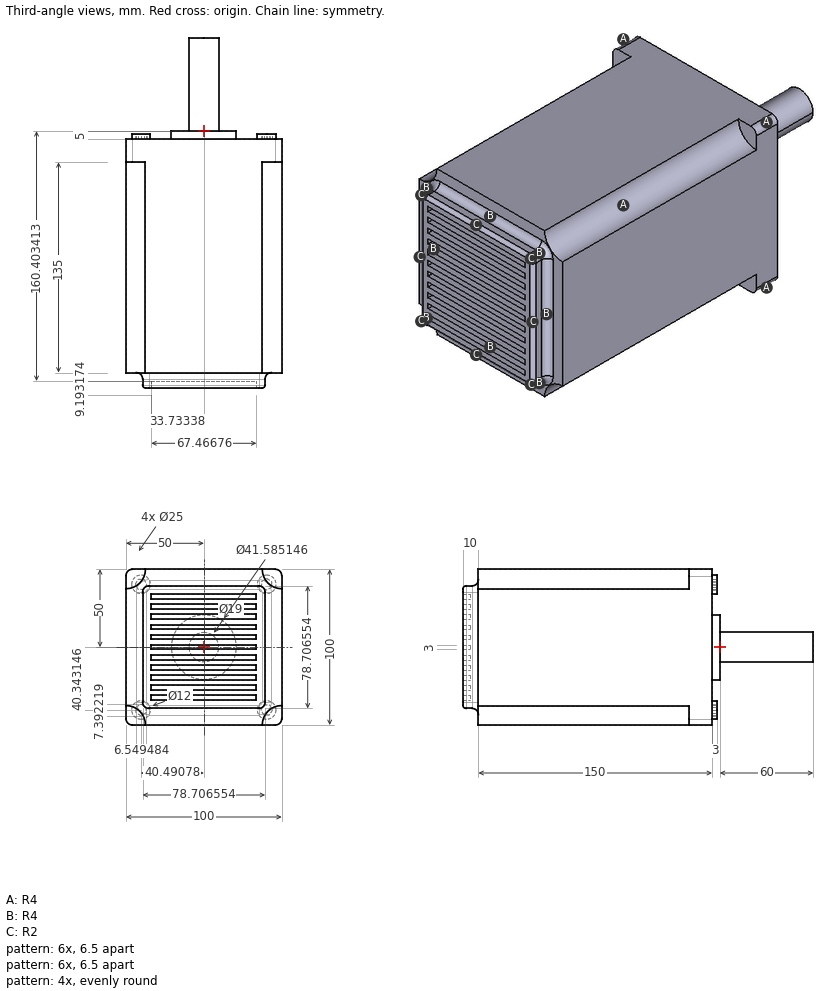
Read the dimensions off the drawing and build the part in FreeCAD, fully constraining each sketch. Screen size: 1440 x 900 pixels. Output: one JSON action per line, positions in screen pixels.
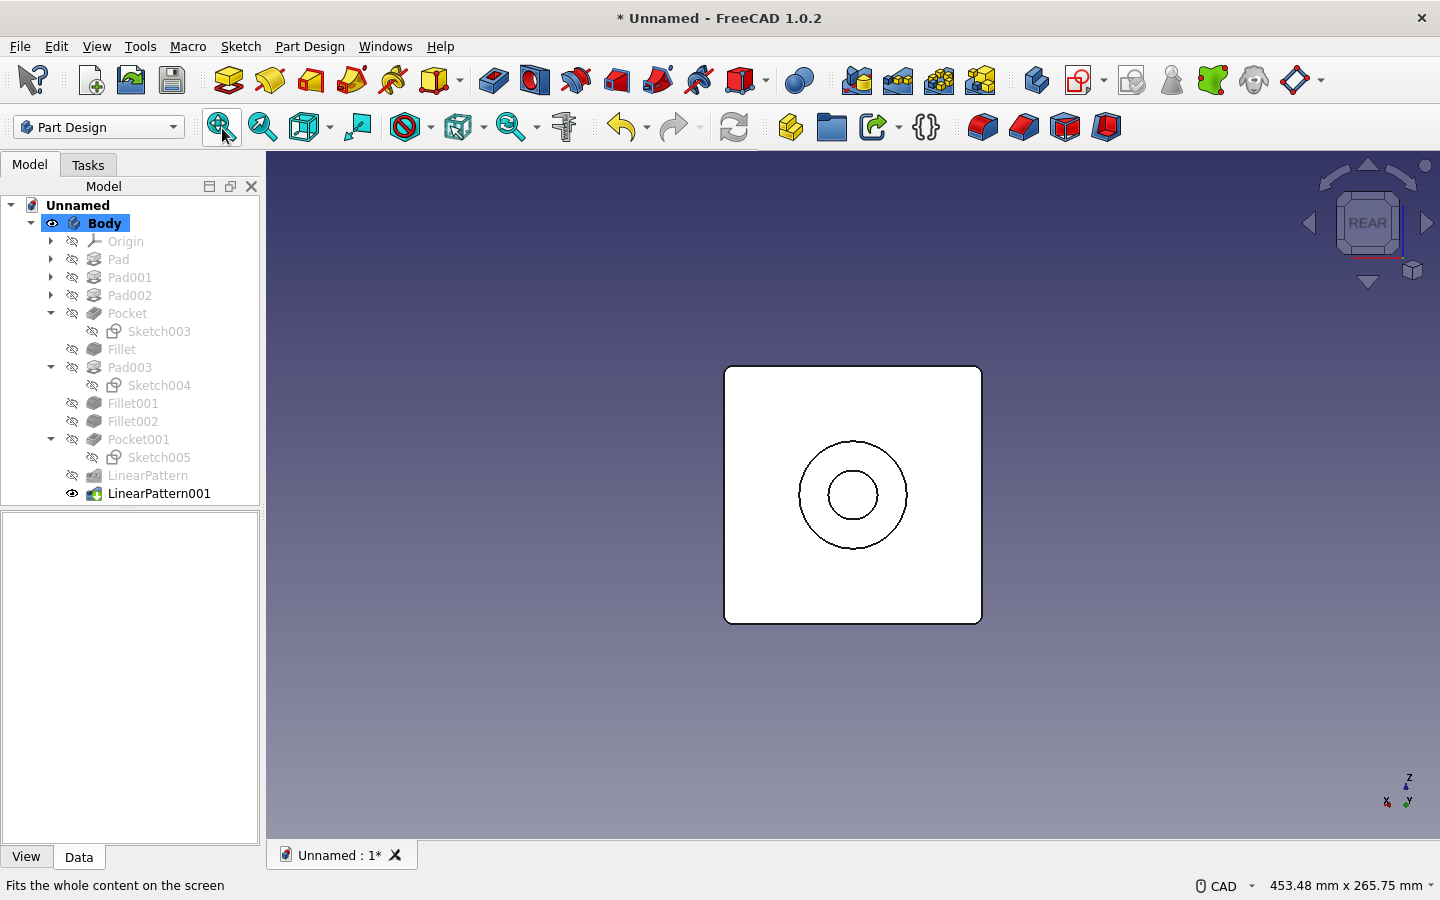
{"action": "left_click", "coordinate": [779, 568]}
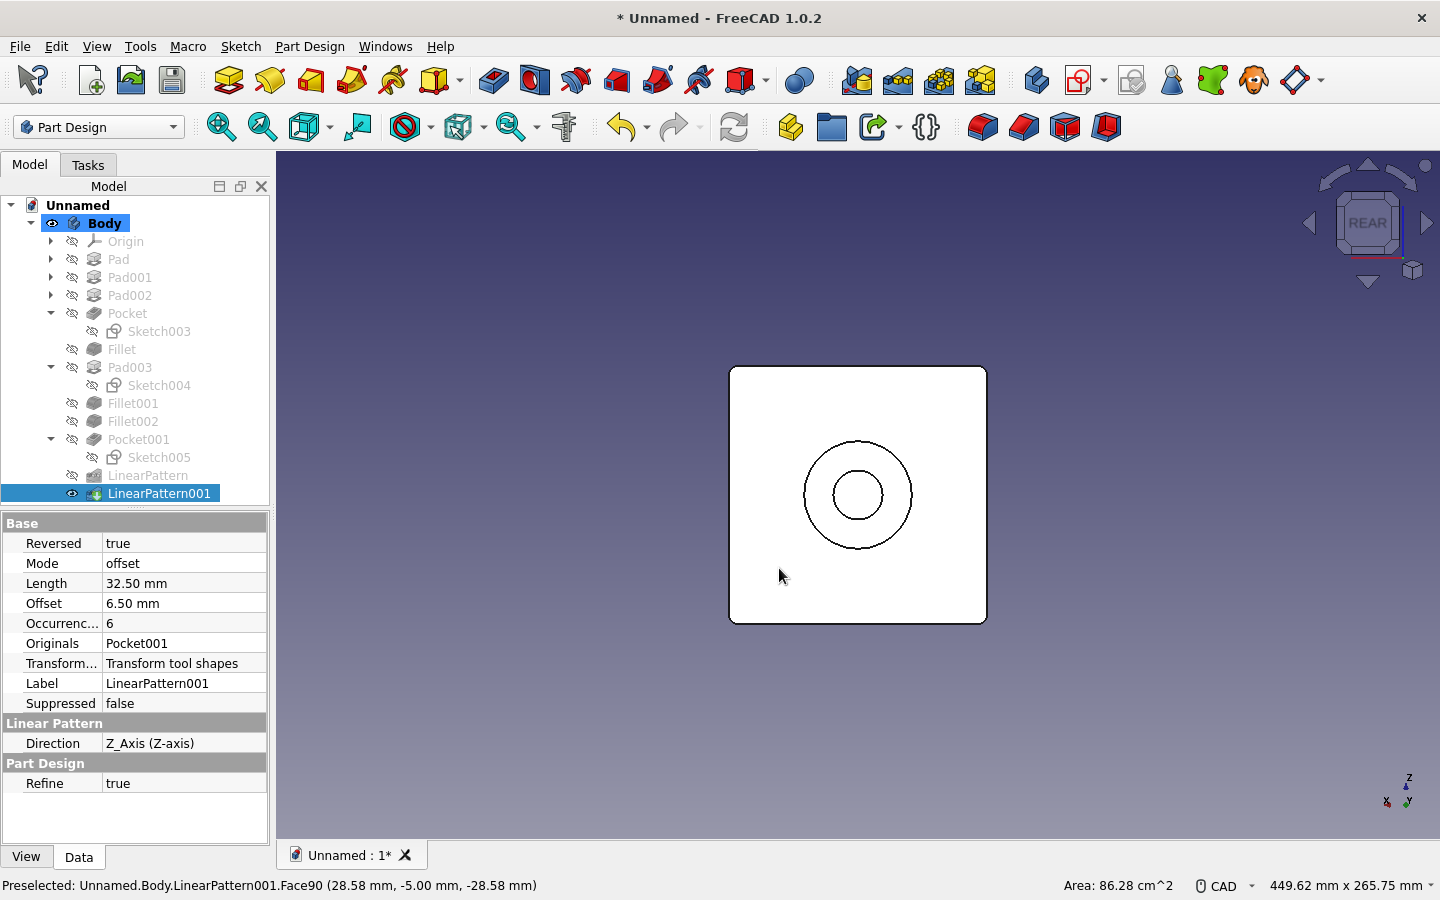
{"action": "left_click", "coordinate": [1078, 80]}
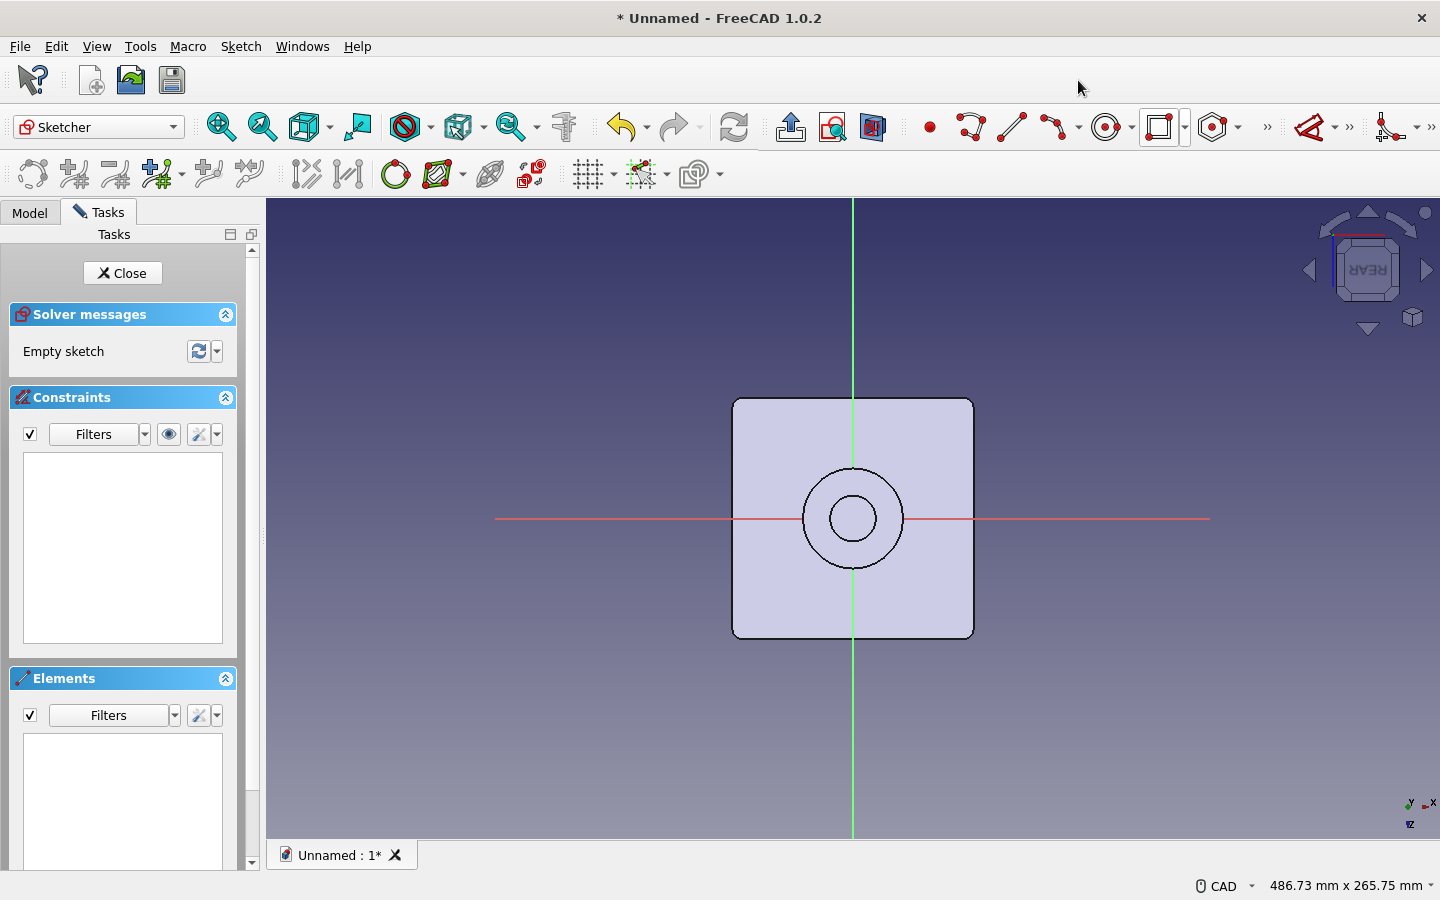
{"action": "scroll", "coordinate": [753, 413], "scroll_direction": "up", "scroll_amount": 13}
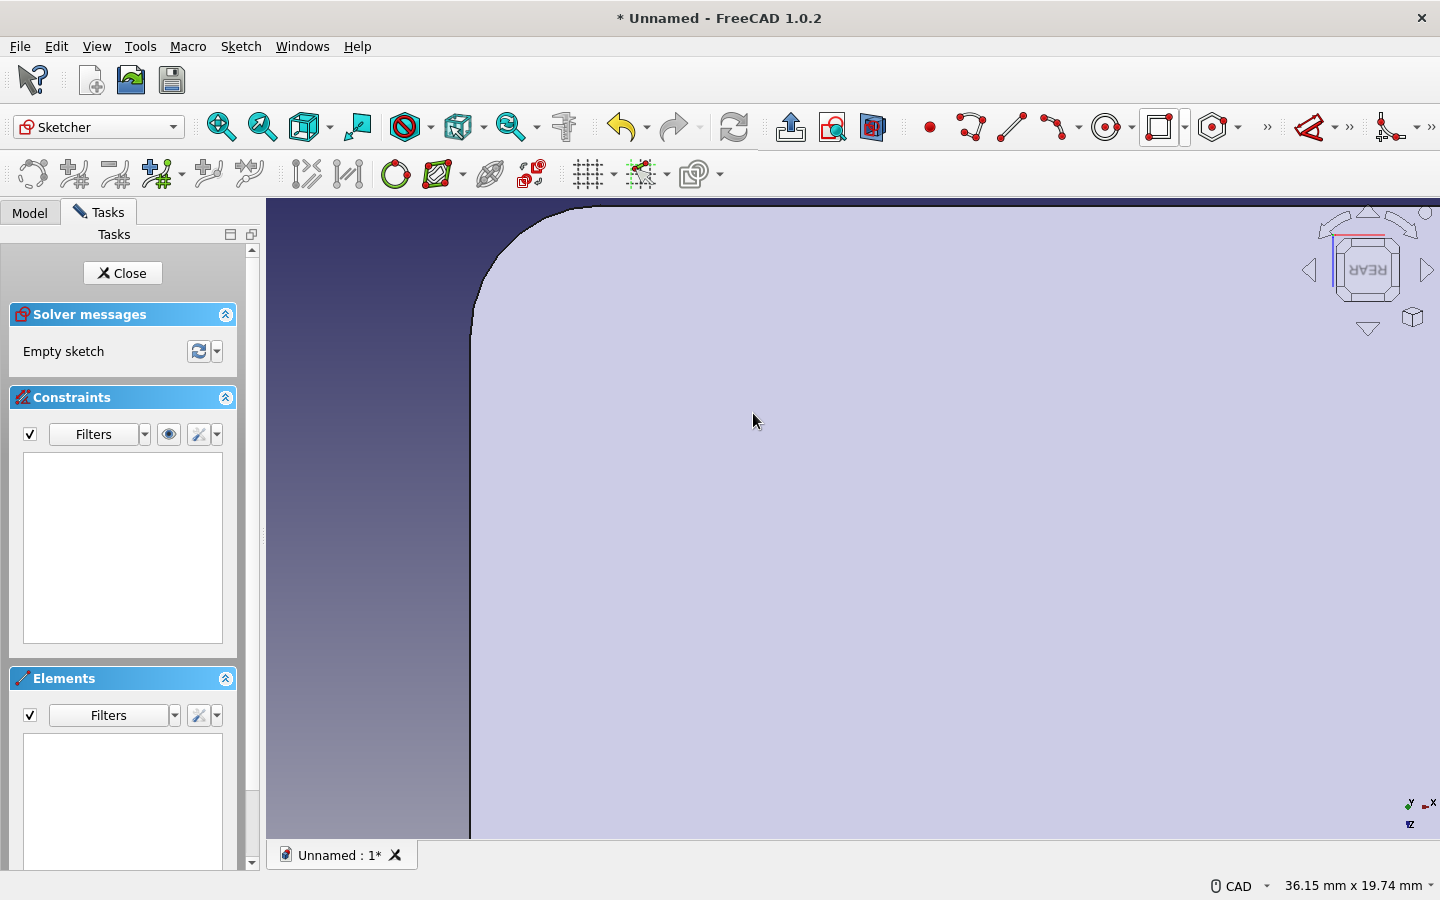
{"action": "left_click", "coordinate": [1212, 128]}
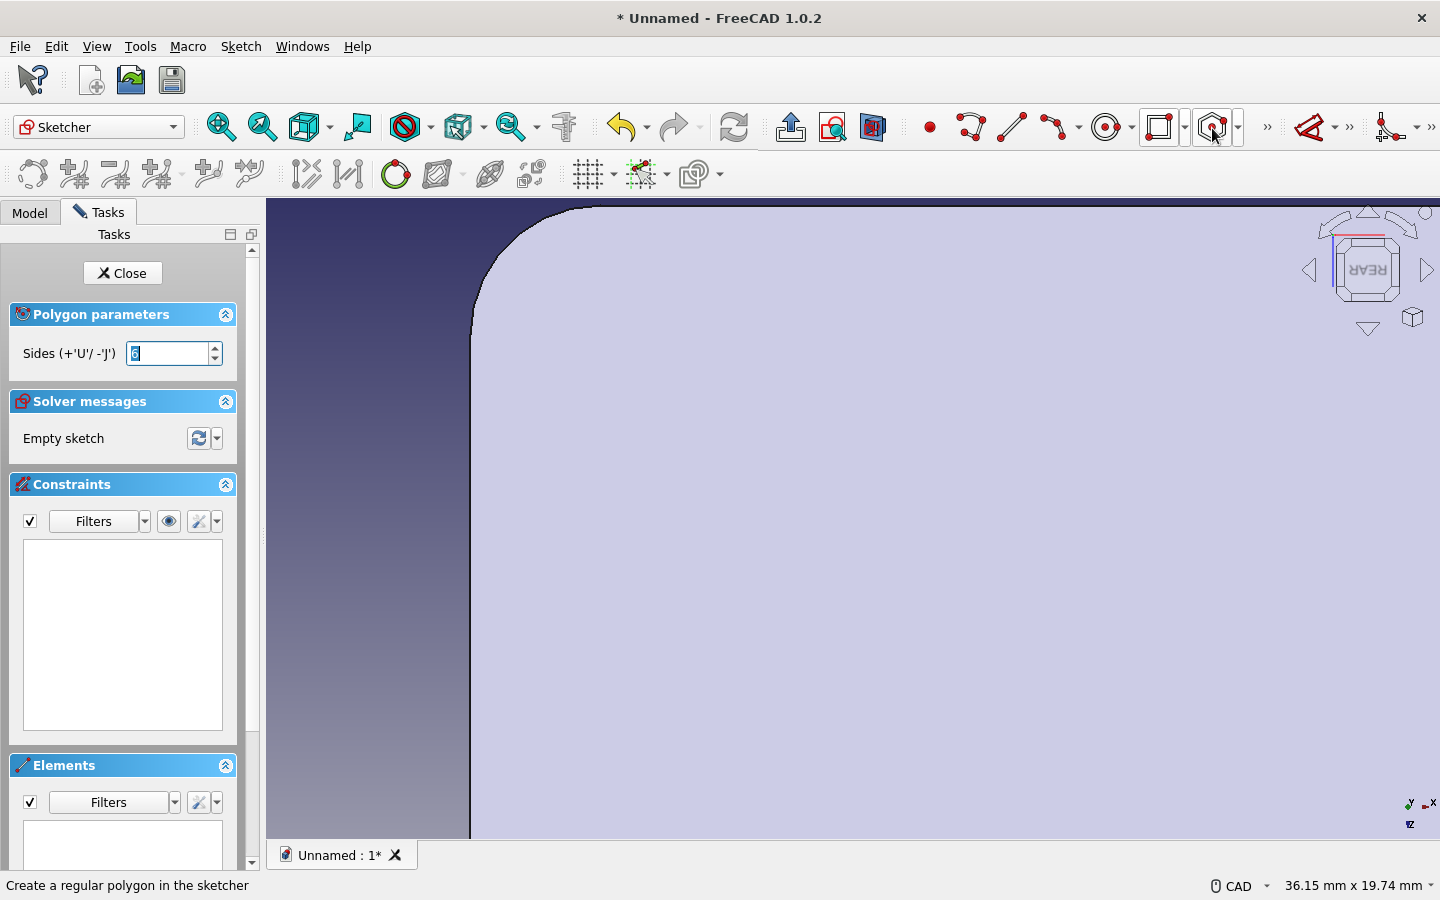
{"action": "left_click", "coordinate": [784, 519]}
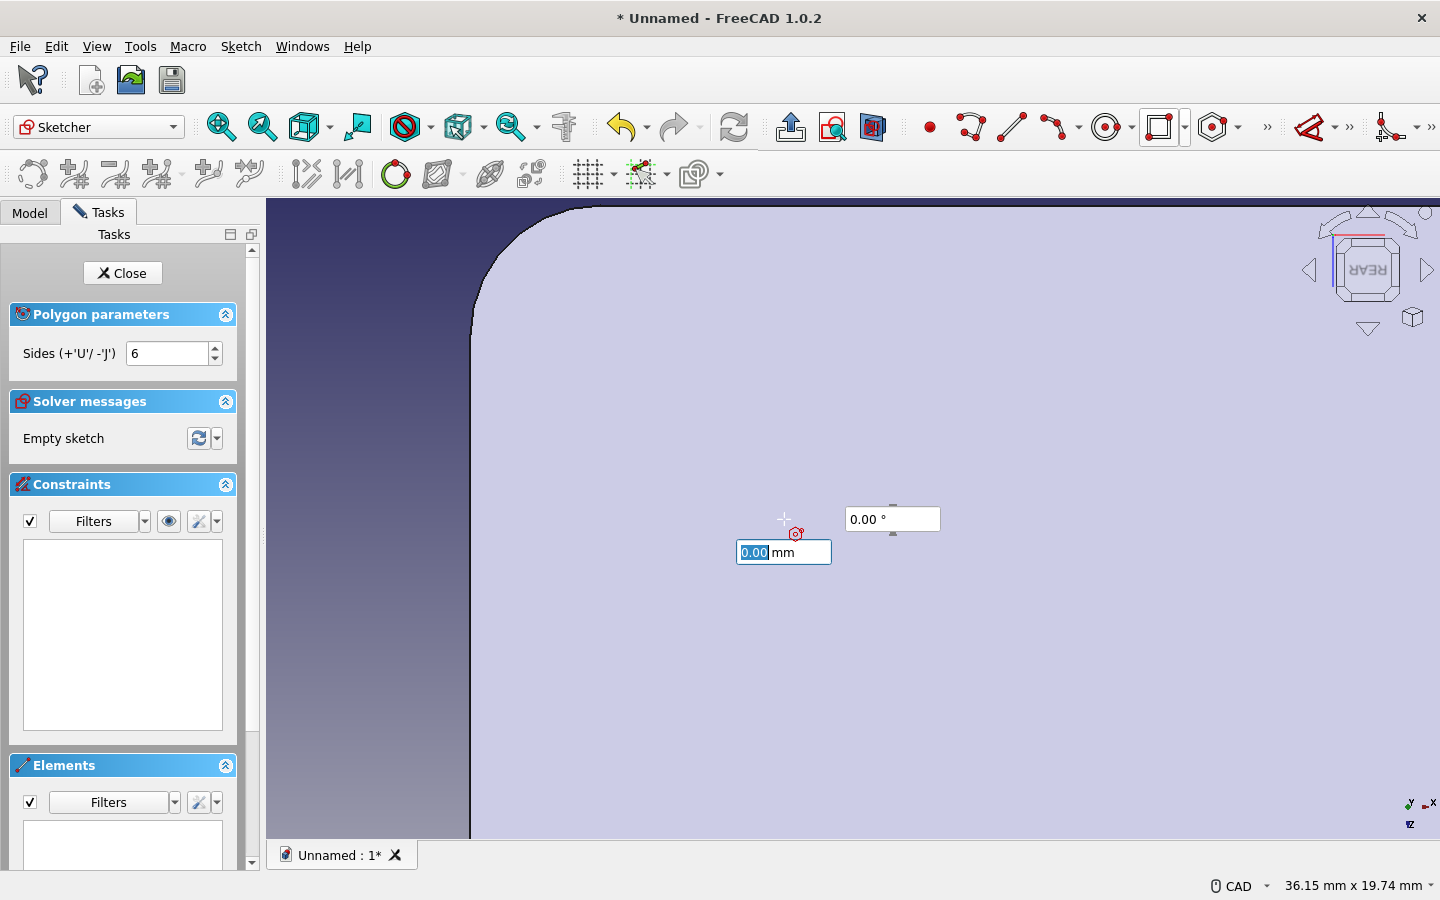
{"action": "left_click", "coordinate": [678, 463]}
{"action": "right_click", "coordinate": [678, 463]}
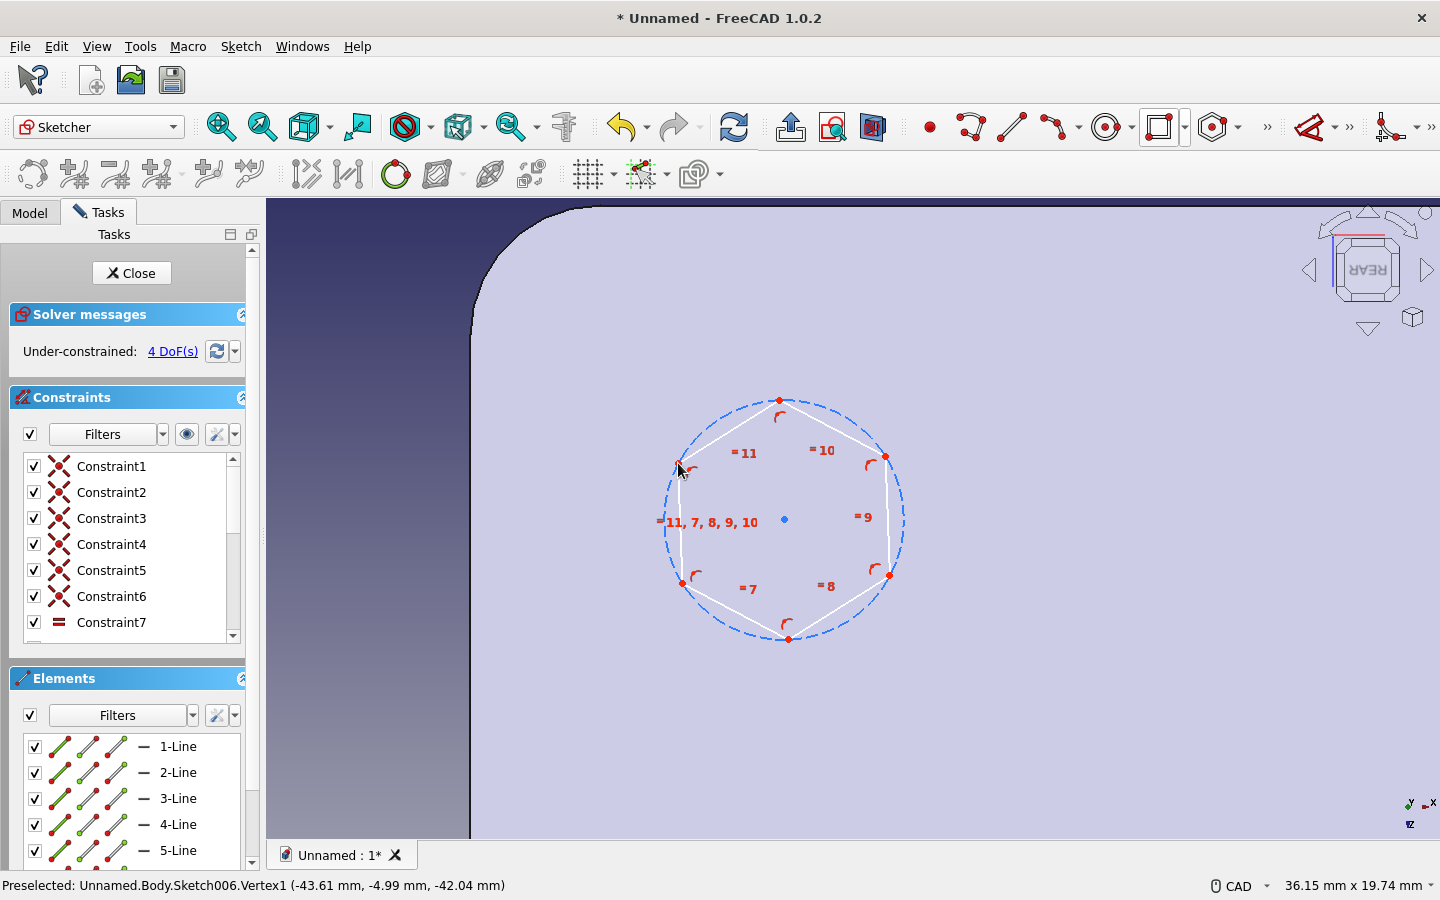
{"action": "left_click", "coordinate": [1106, 128]}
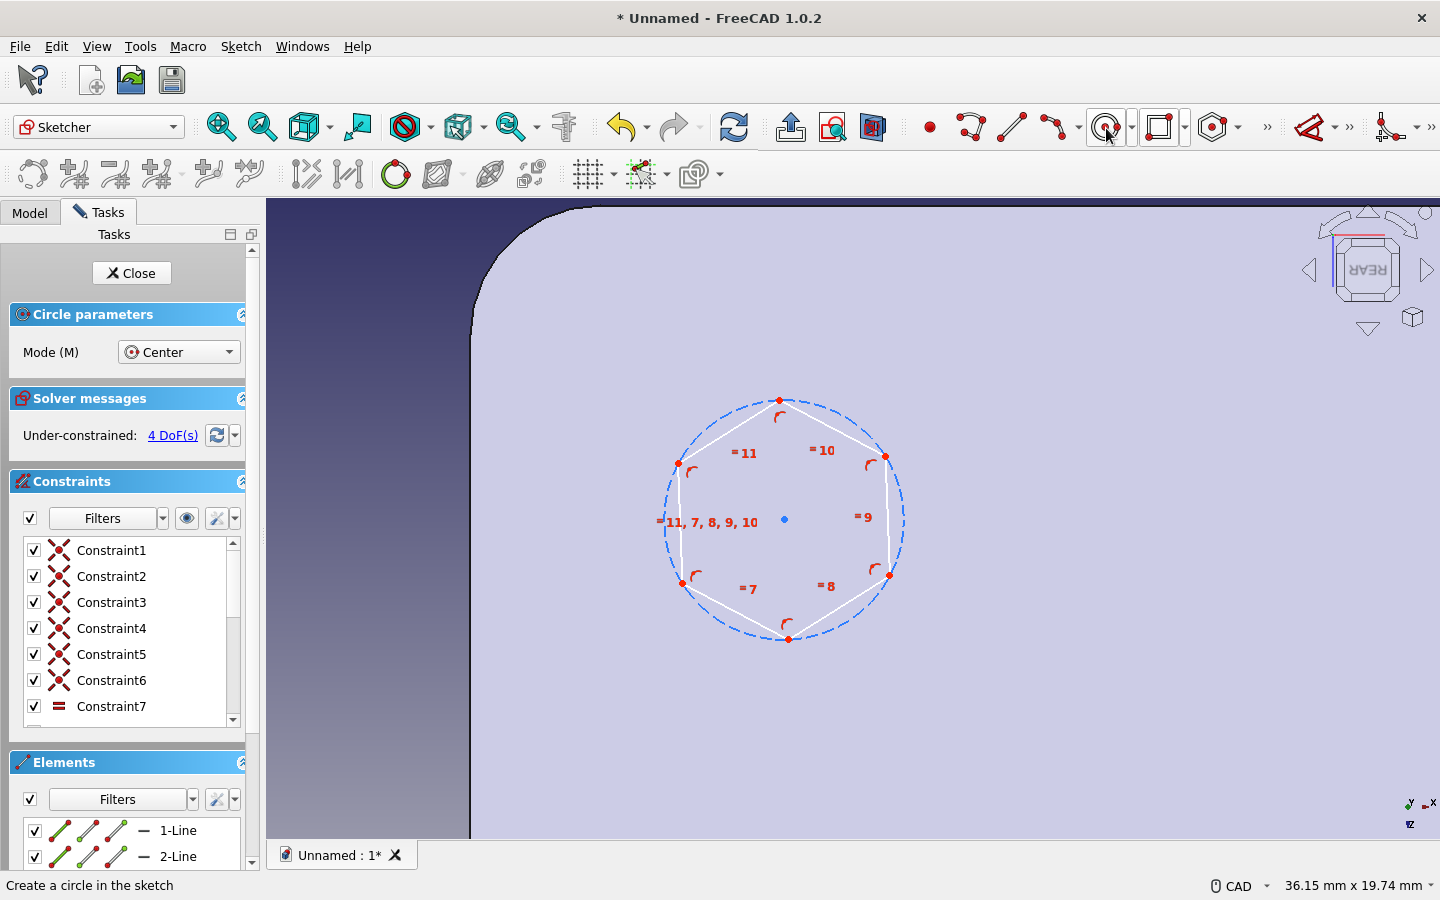
{"action": "left_click", "coordinate": [784, 520]}
{"action": "left_click", "coordinate": [922, 381]}
{"action": "key", "text": "Escape"}